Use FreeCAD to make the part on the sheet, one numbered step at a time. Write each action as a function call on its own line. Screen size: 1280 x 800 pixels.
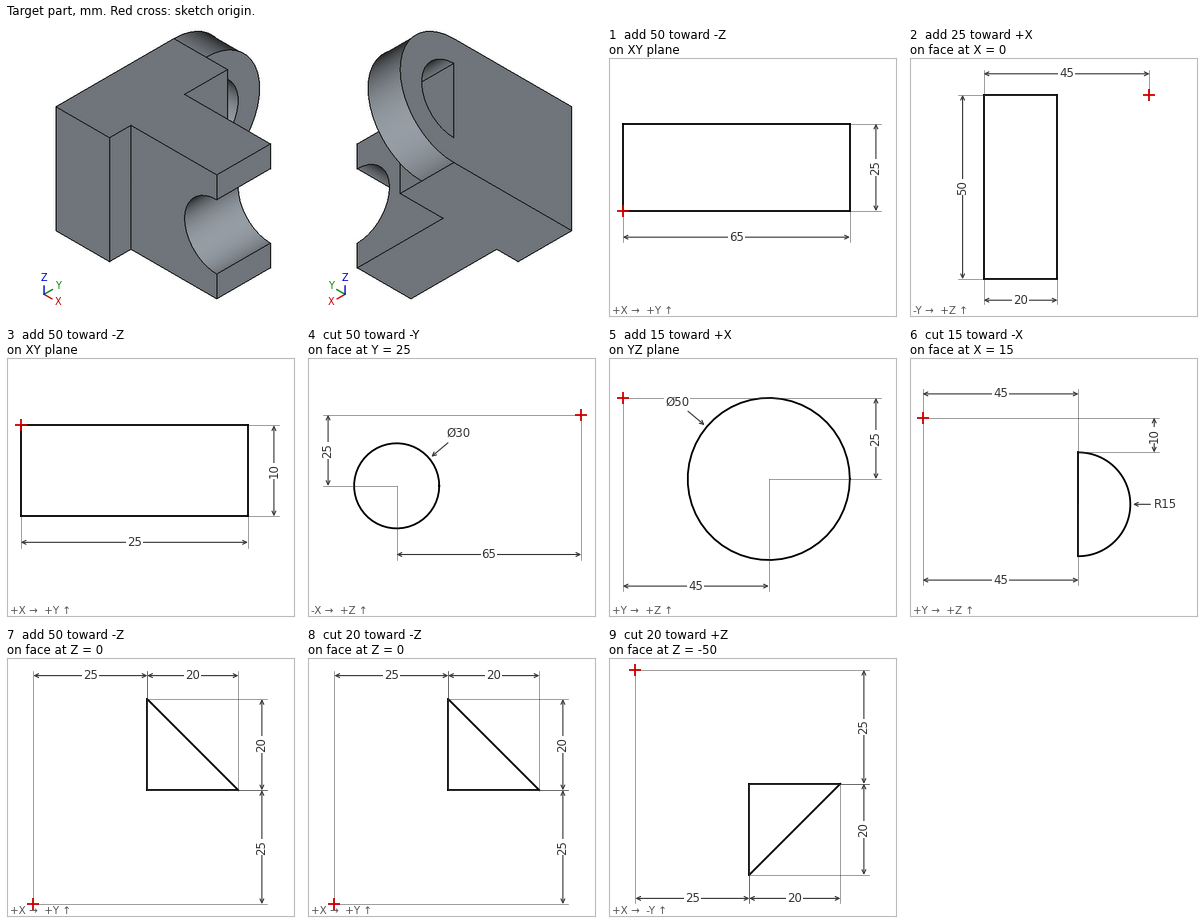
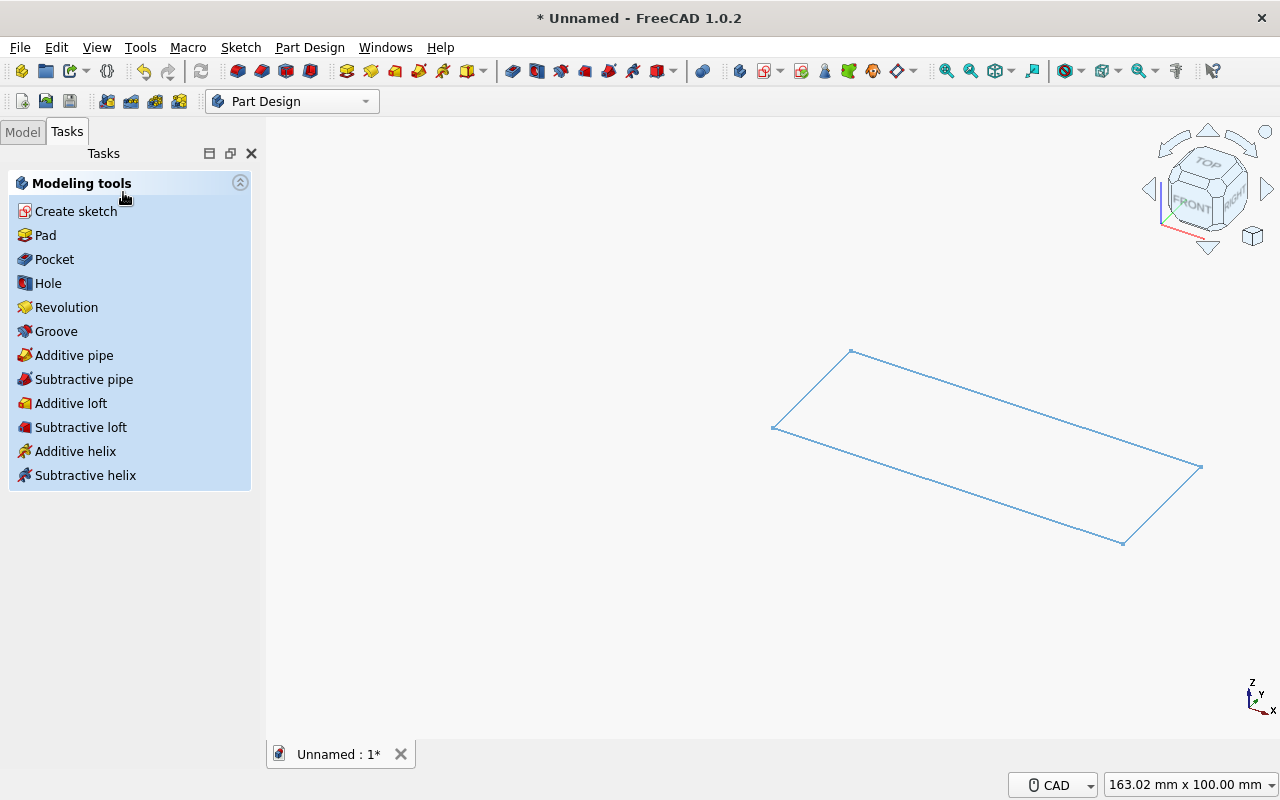
click(348, 72)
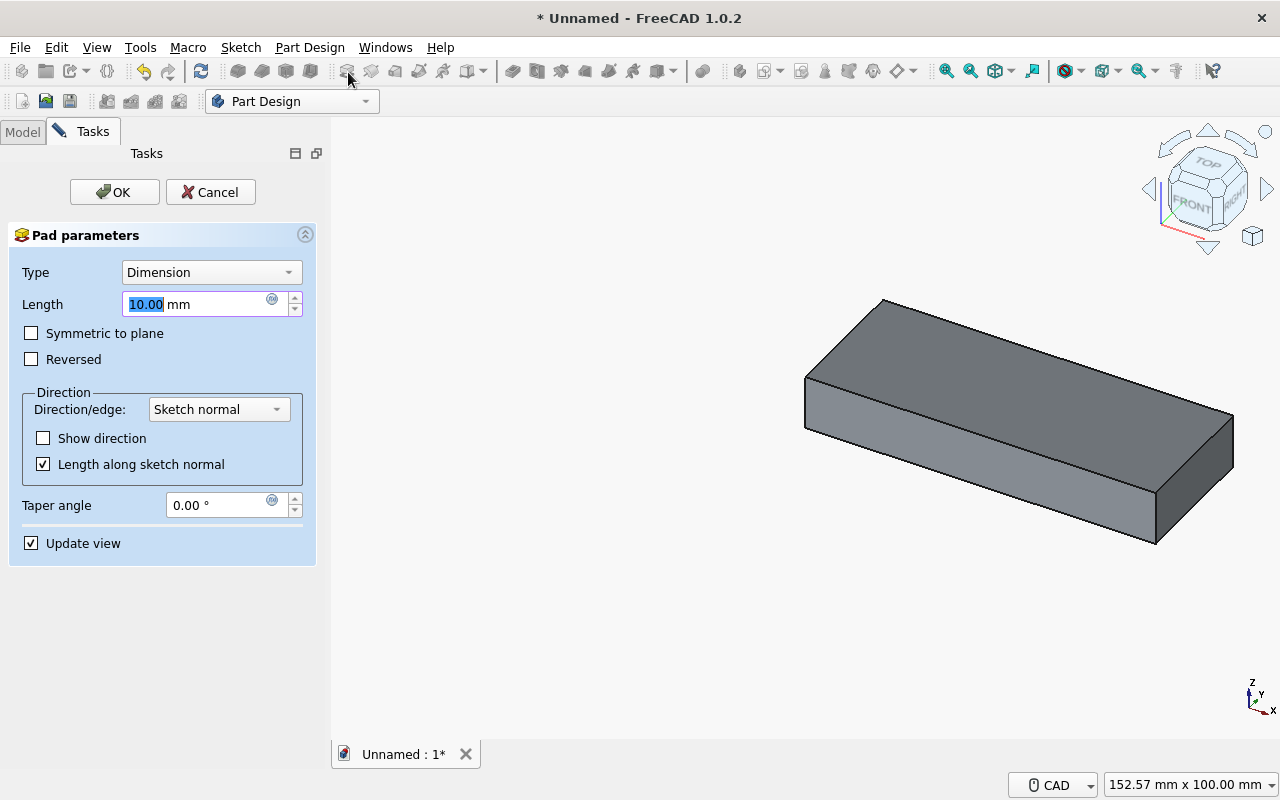
text(50)
key(Tab)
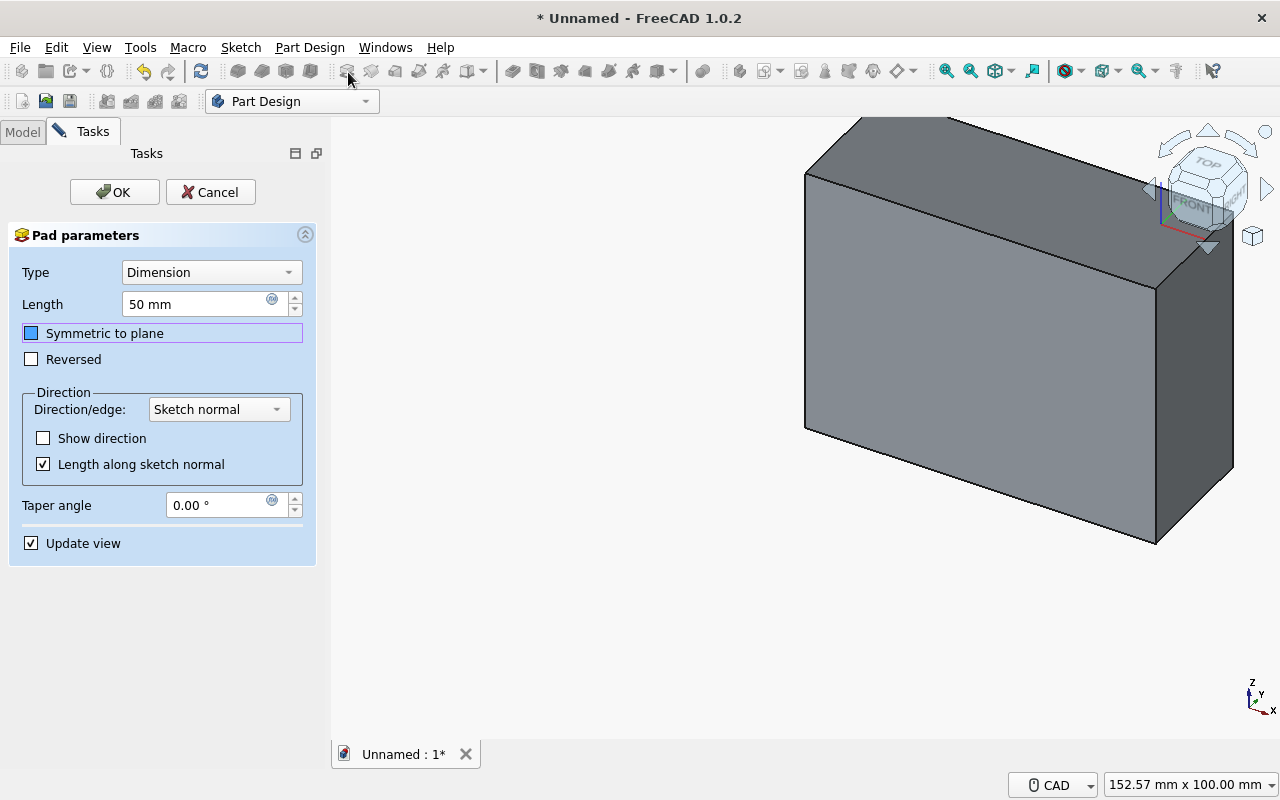
click(30, 359)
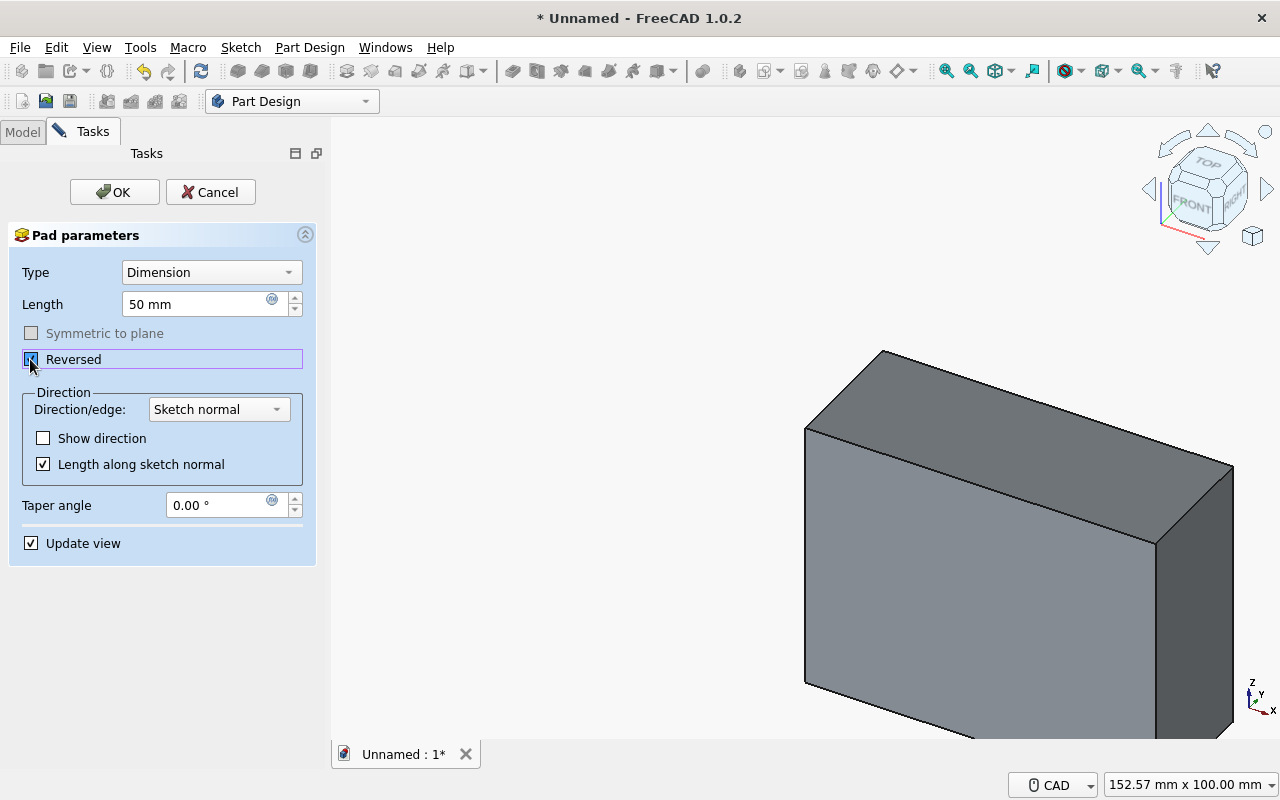
click(115, 192)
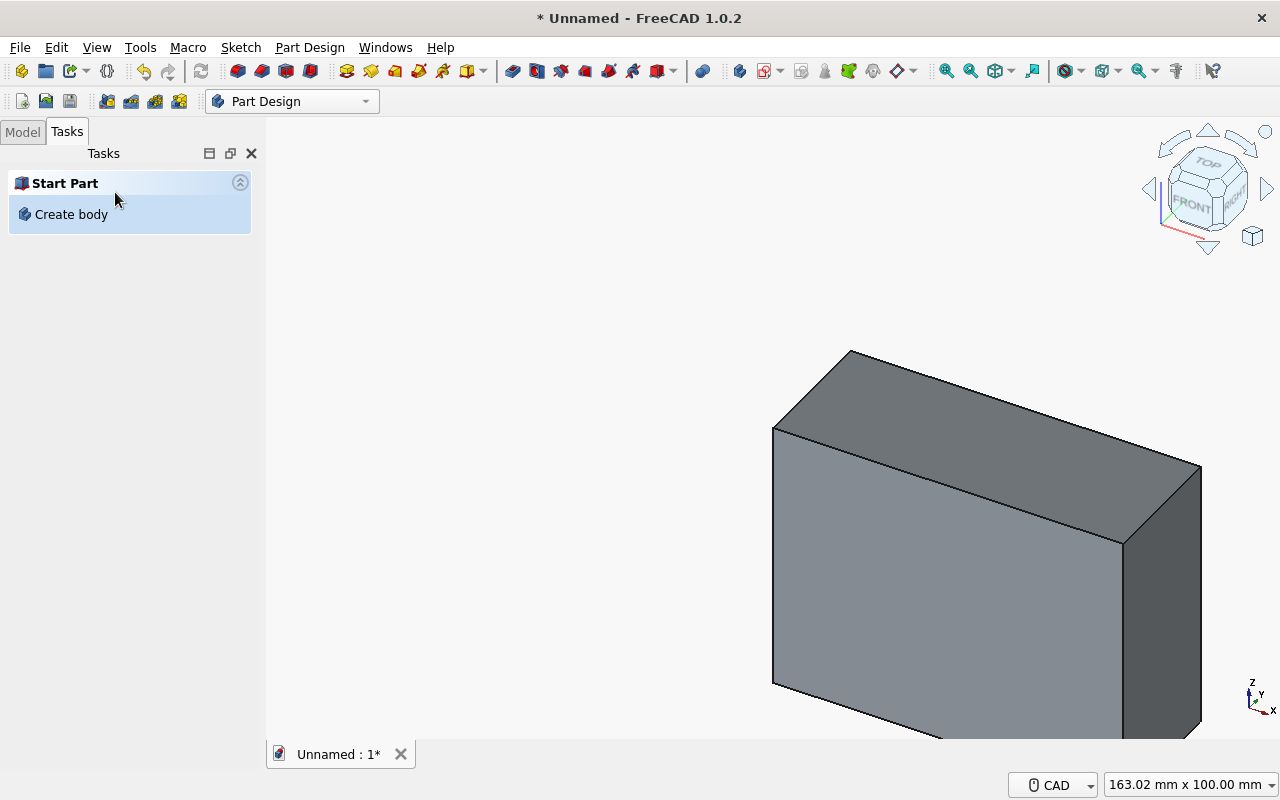
click(948, 72)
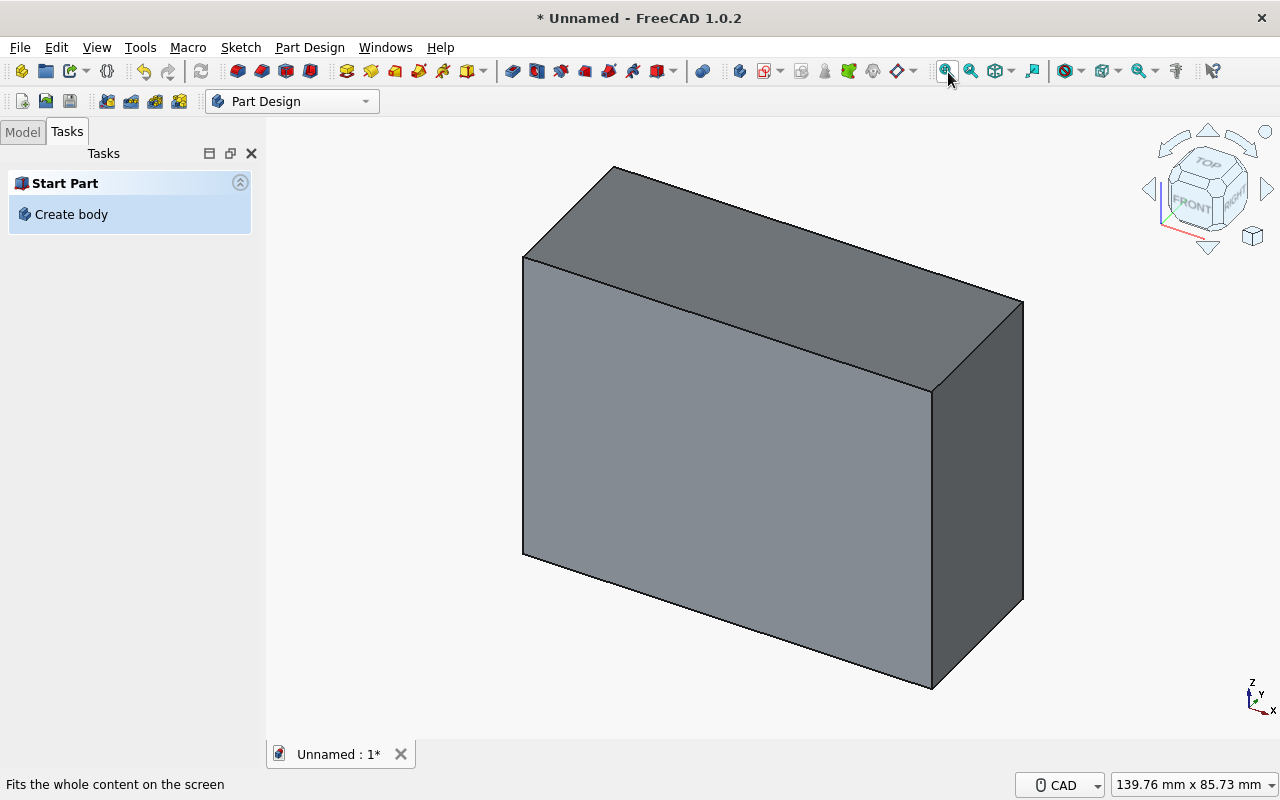
key(6)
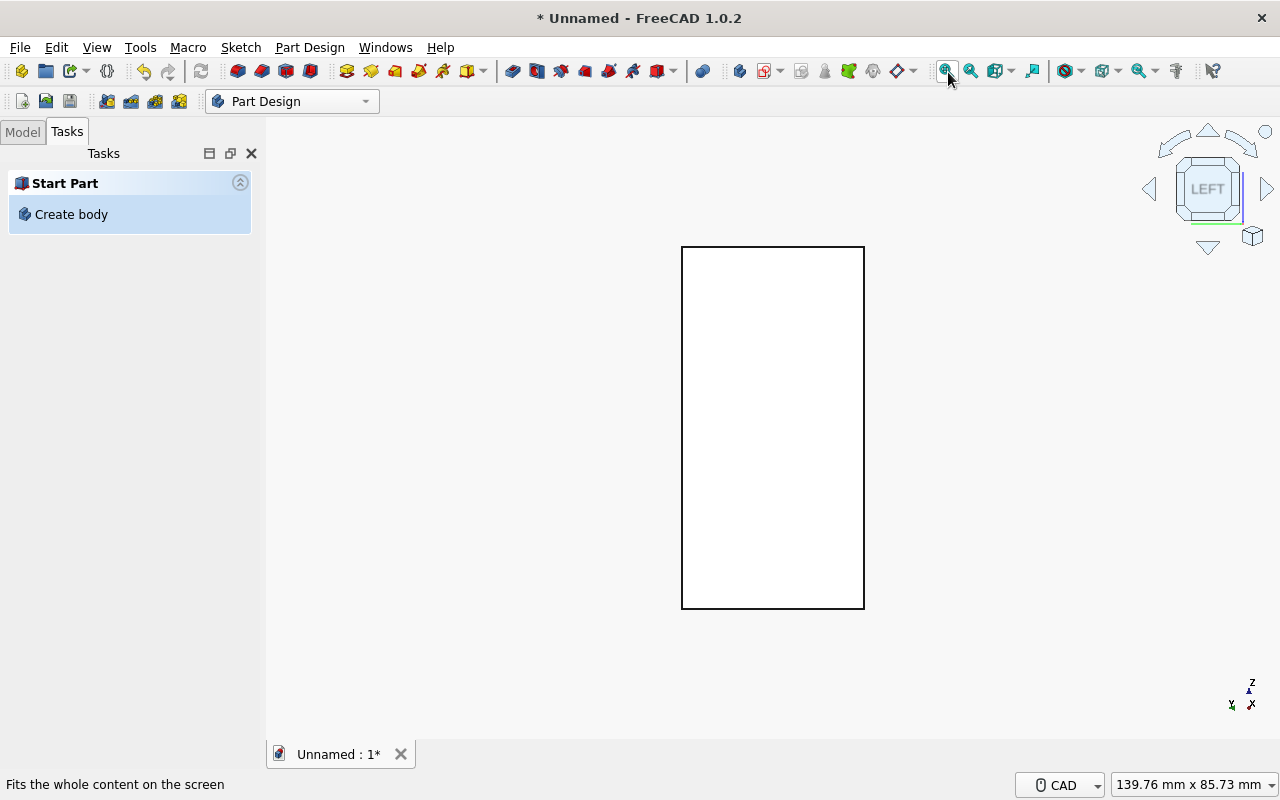
click(773, 375)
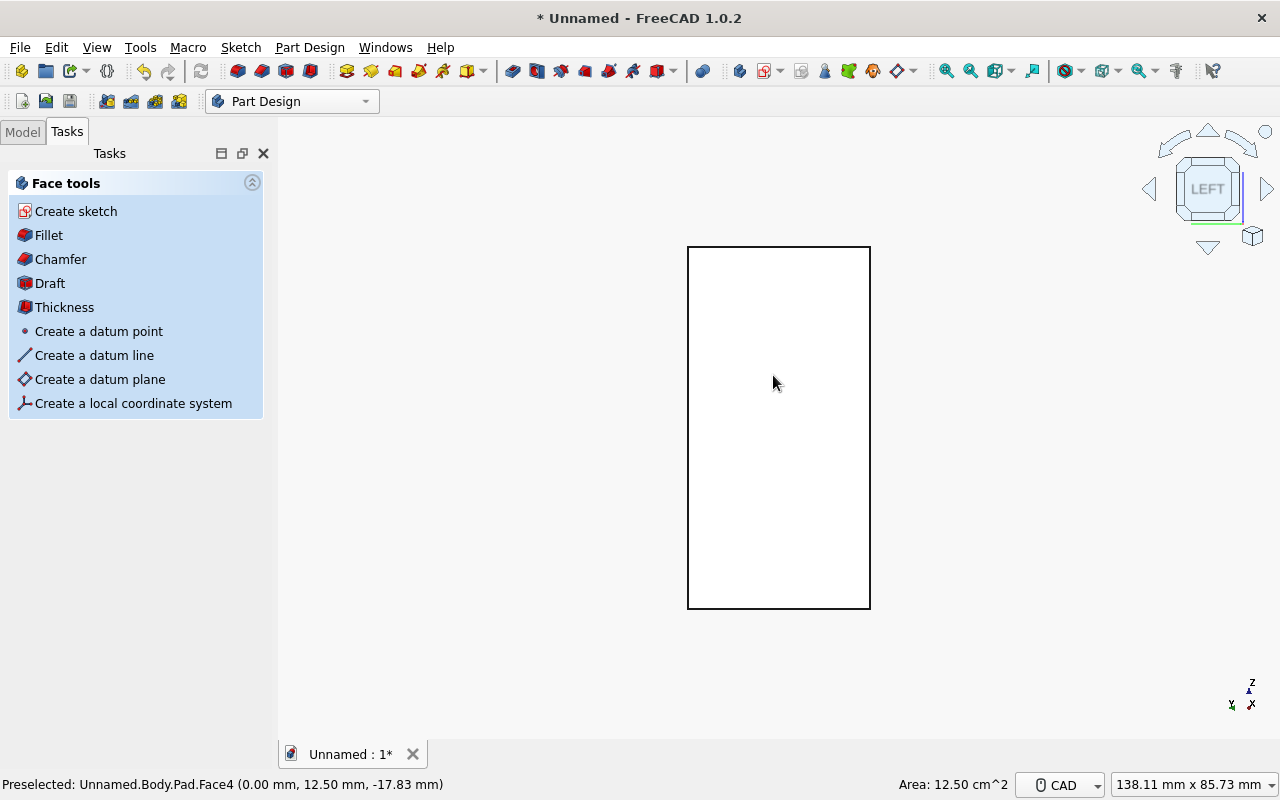
click(764, 72)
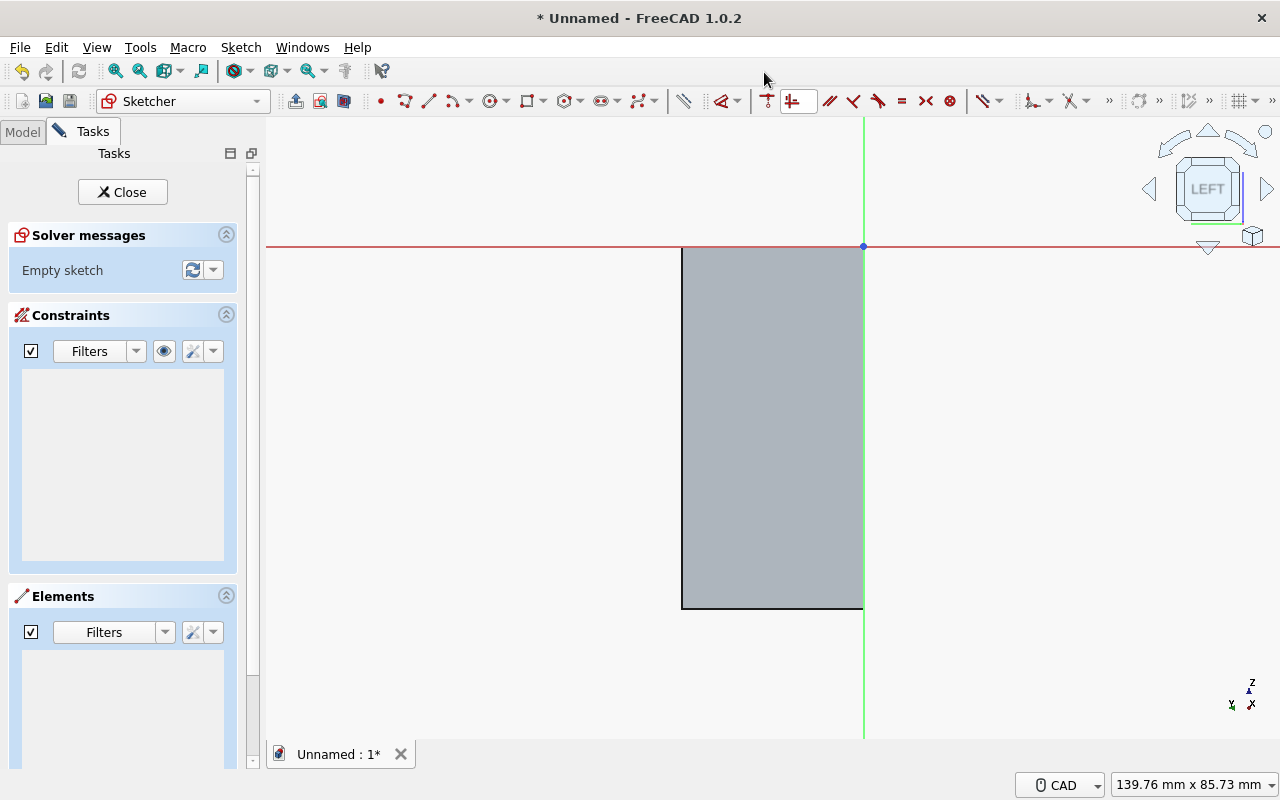
click(528, 102)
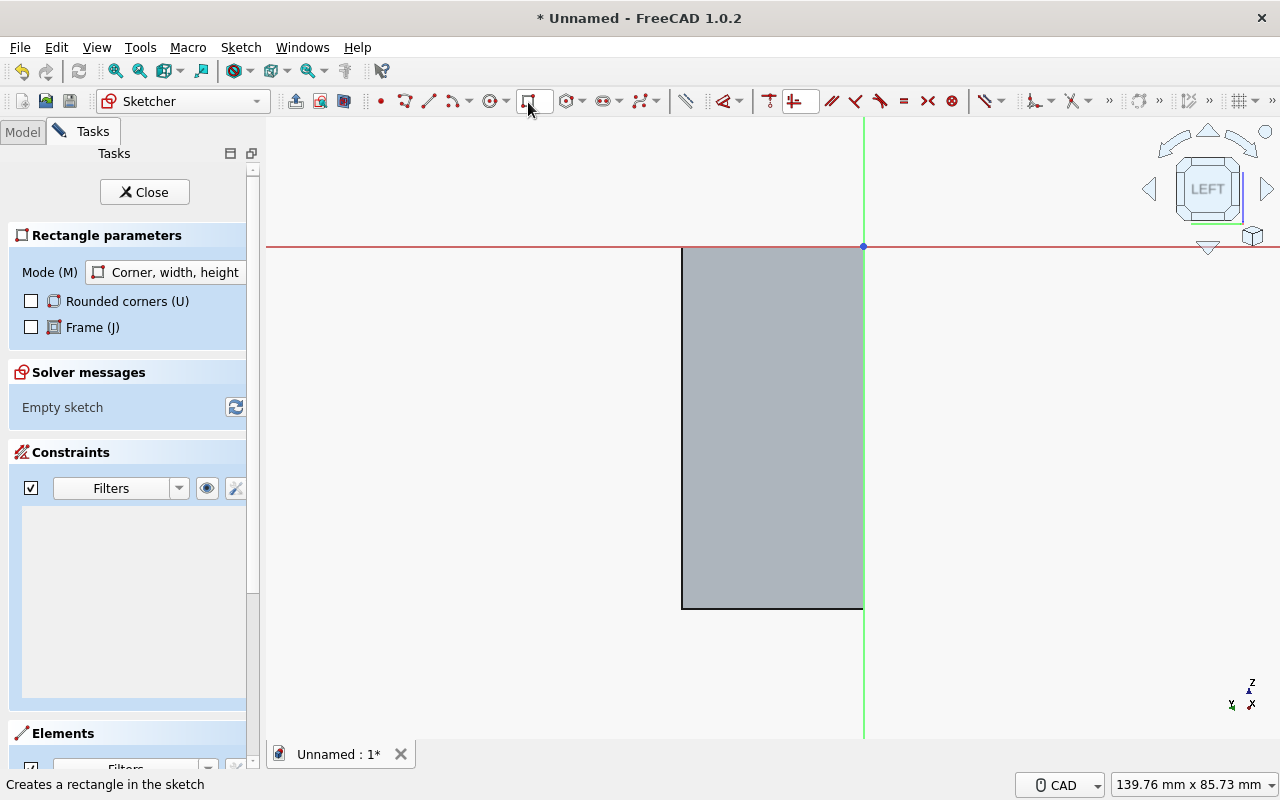
click(537, 247)
move(682, 609)